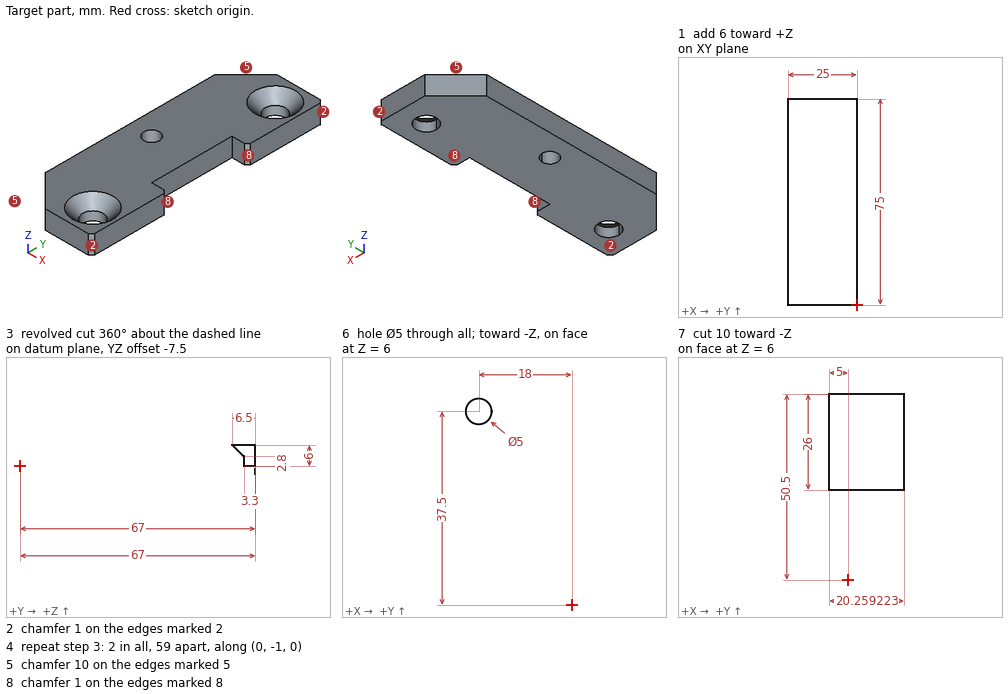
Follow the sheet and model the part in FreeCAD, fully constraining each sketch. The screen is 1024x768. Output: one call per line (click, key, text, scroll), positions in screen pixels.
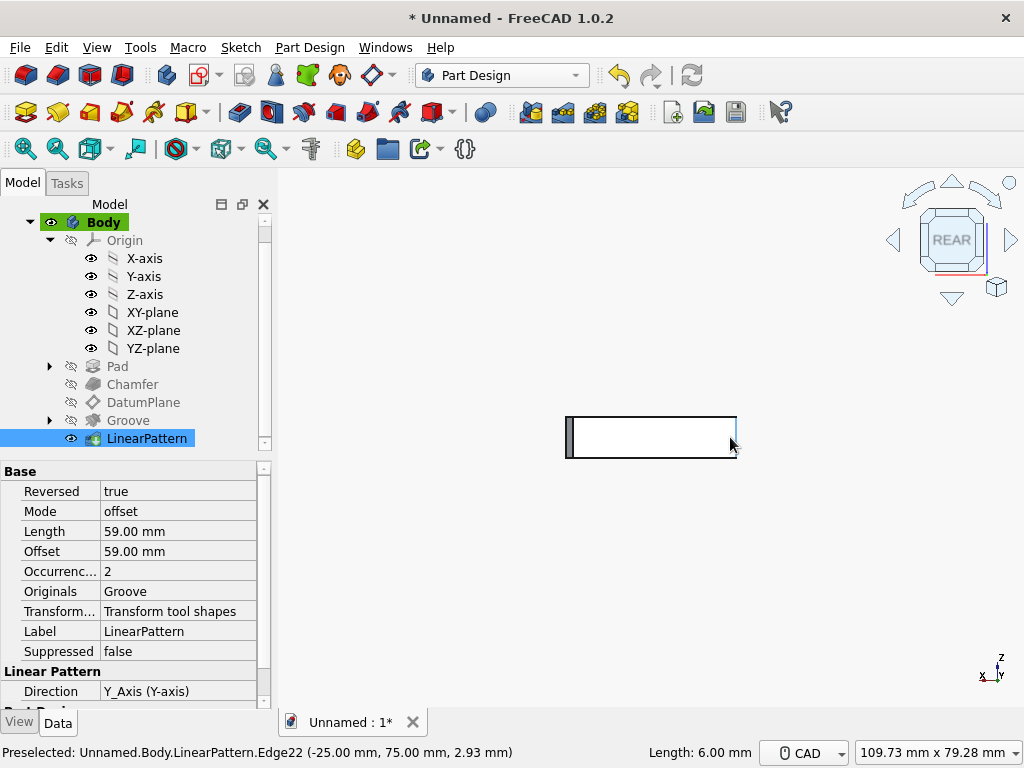
key(6)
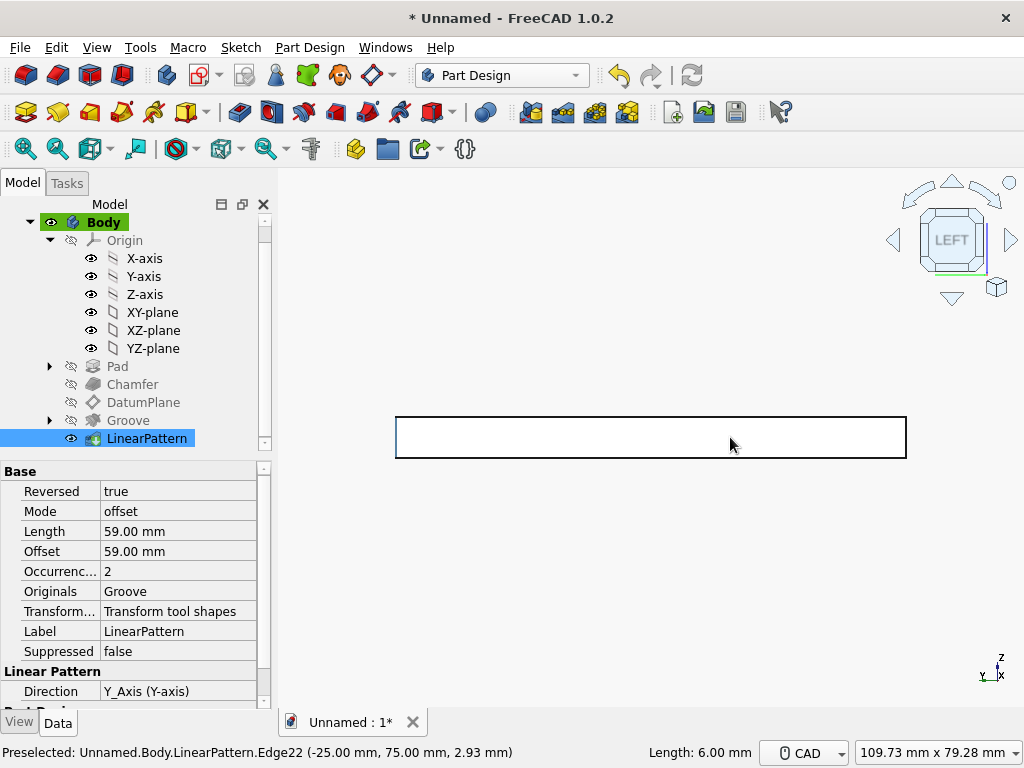
click(906, 436, ctrl)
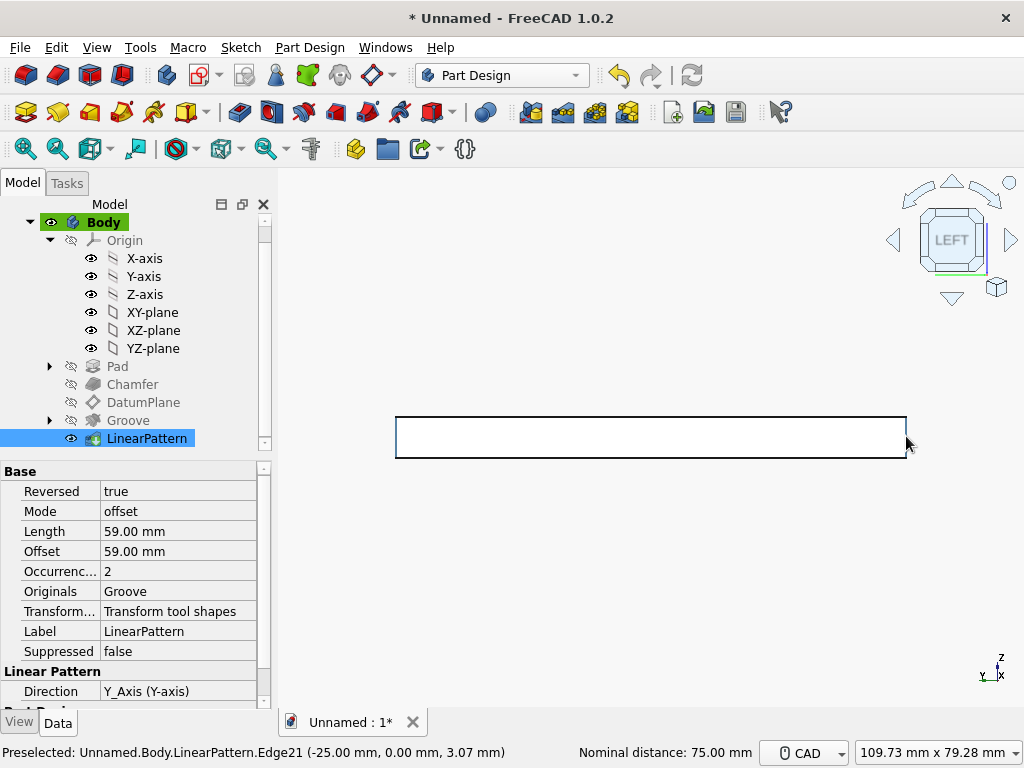
click(58, 76)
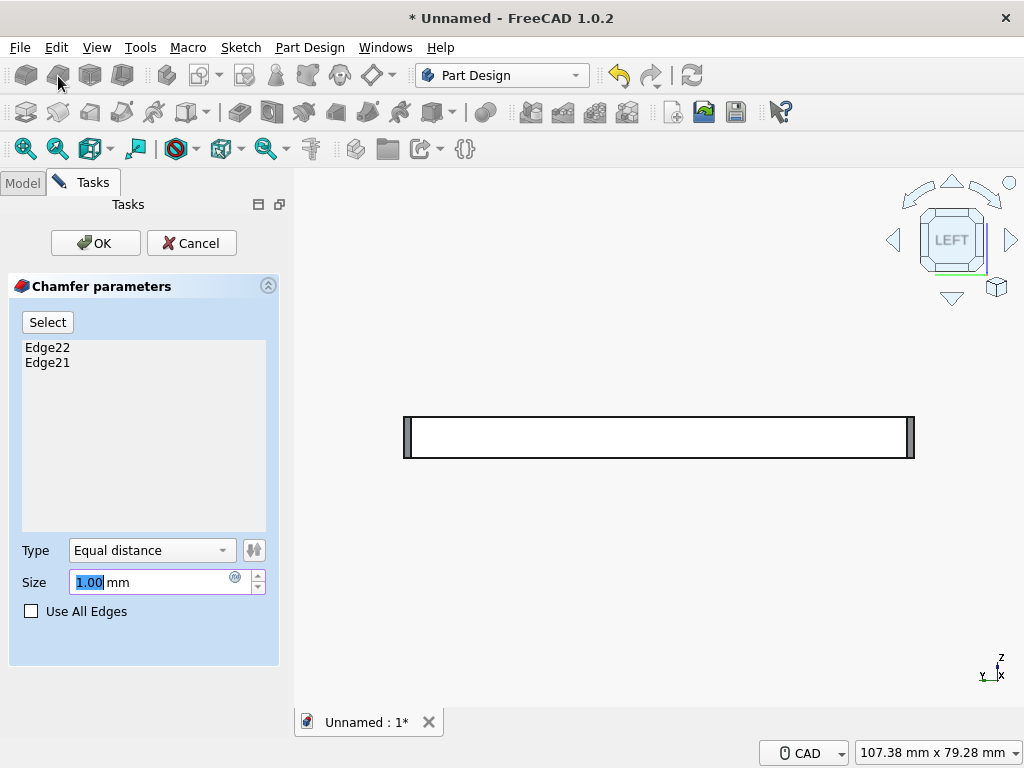
text(10)
key(Tab)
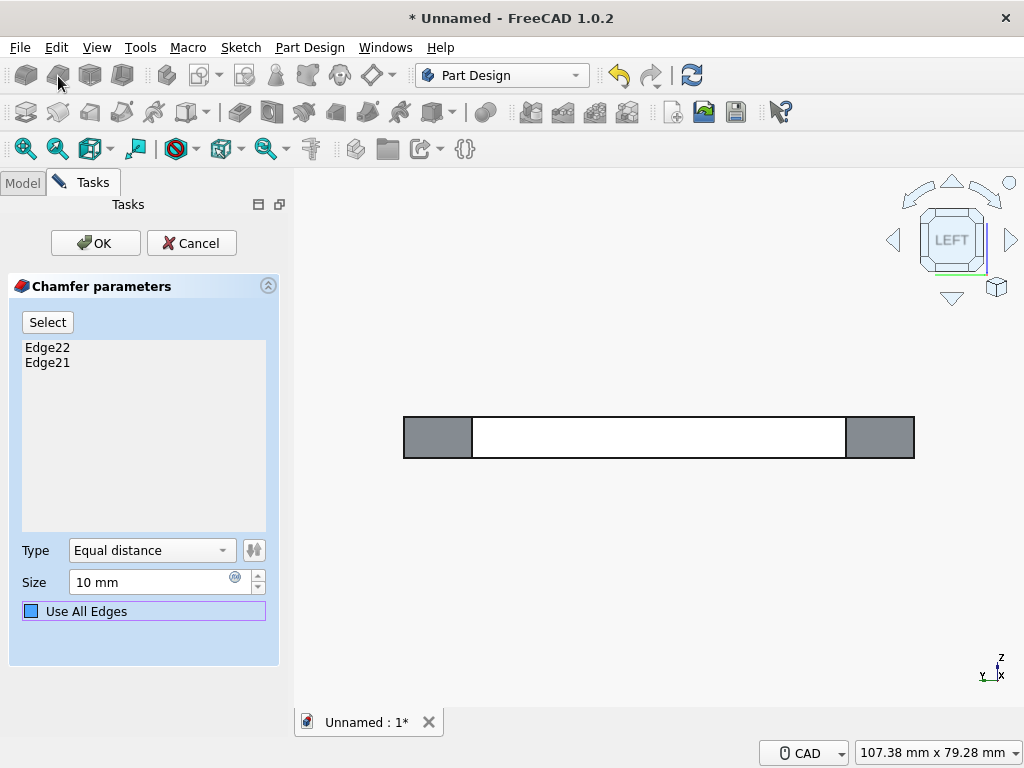
click(96, 243)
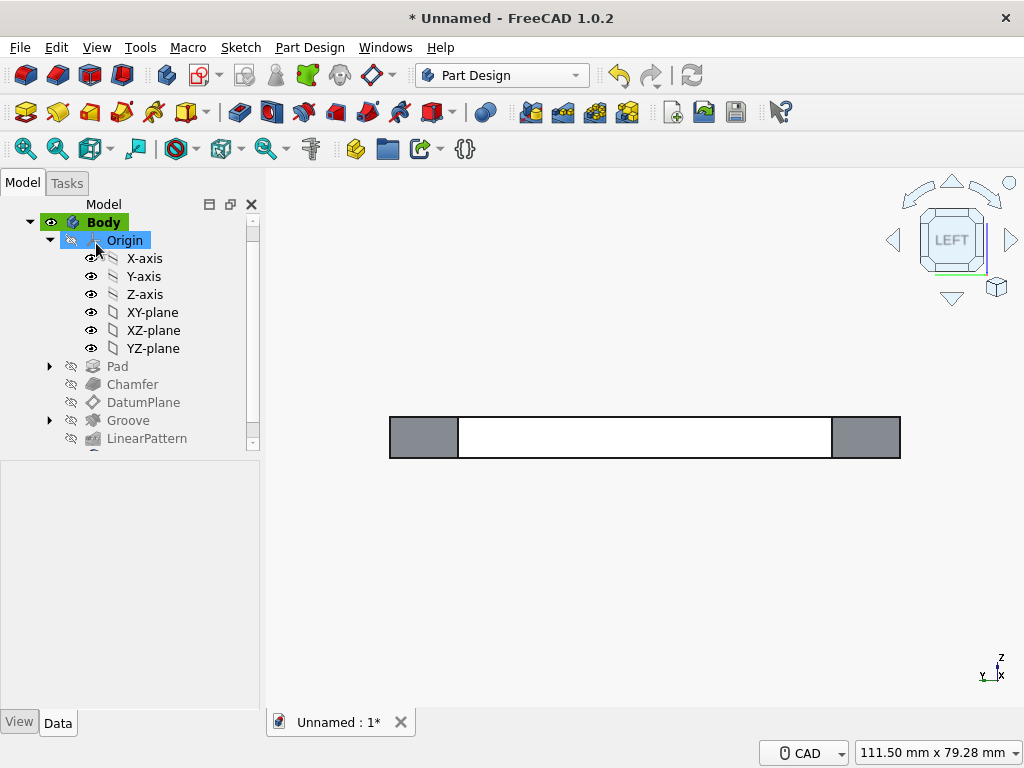
key(0)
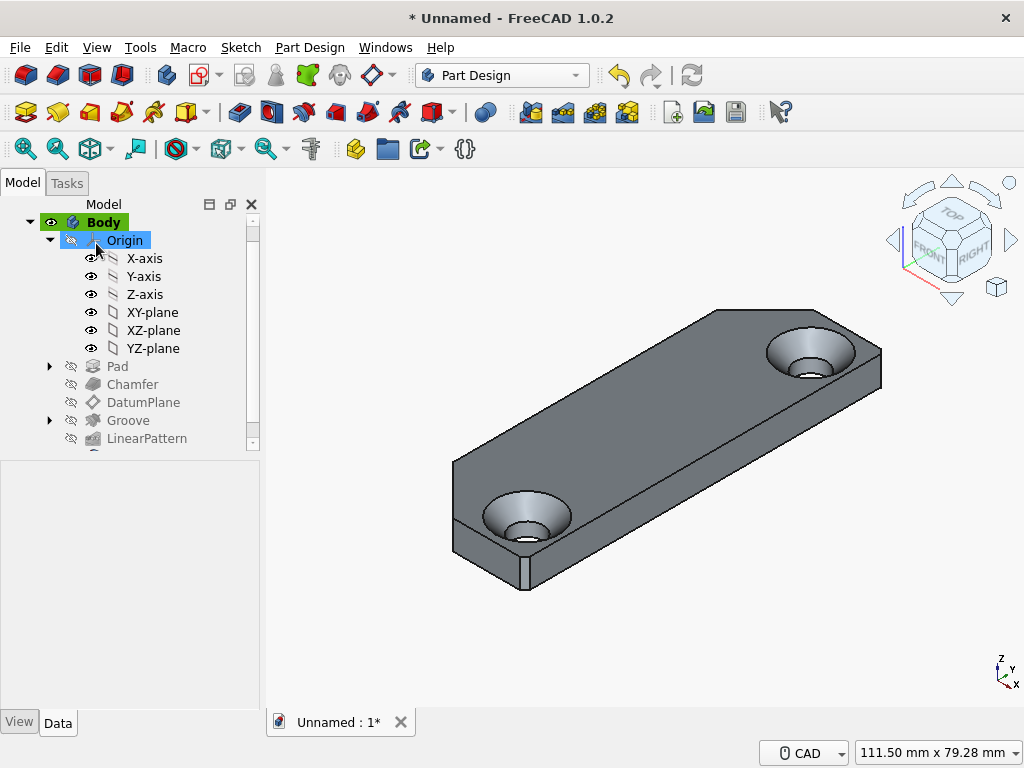
click(697, 390)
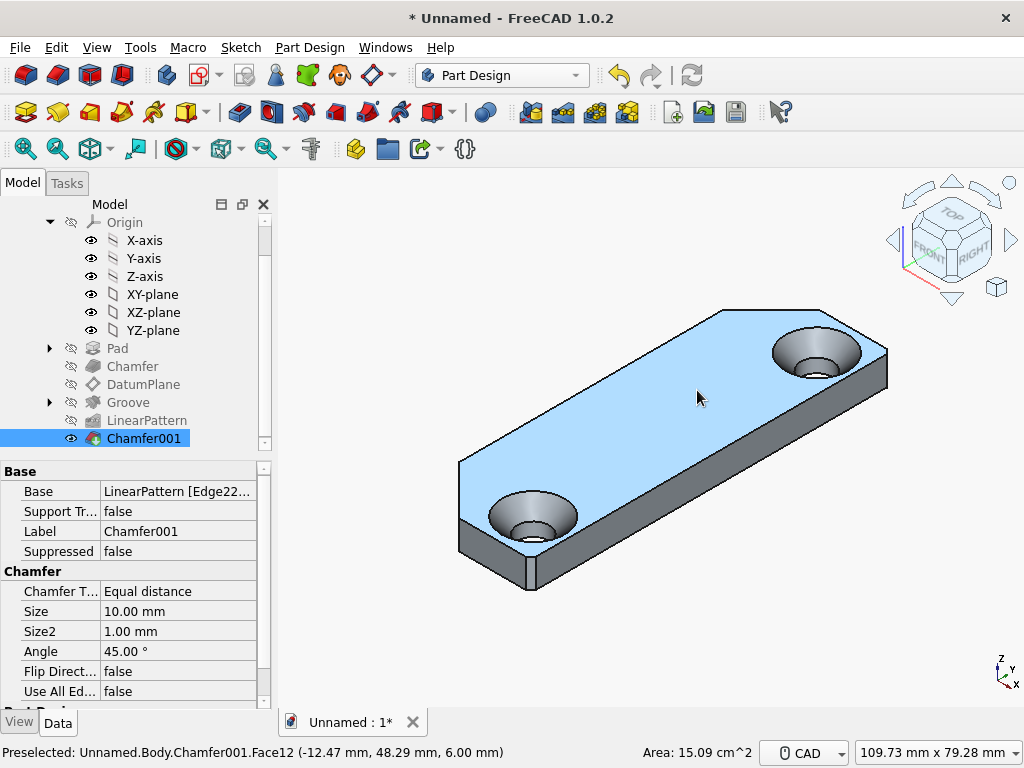
click(200, 76)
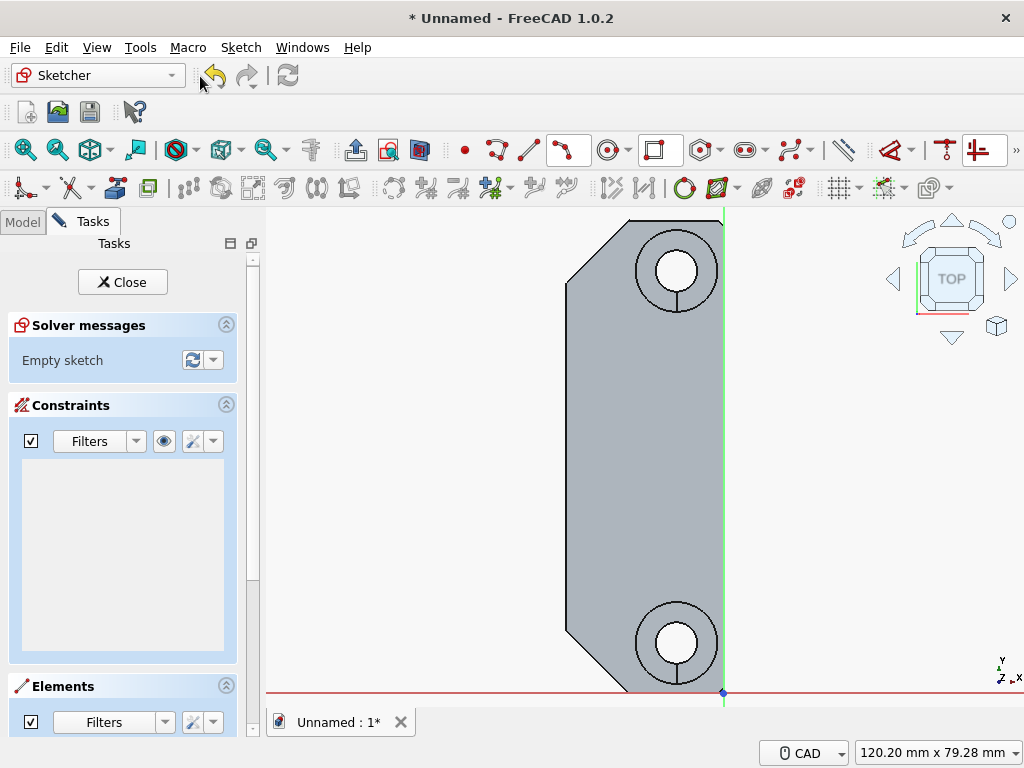
scroll(615, 457, up, 11)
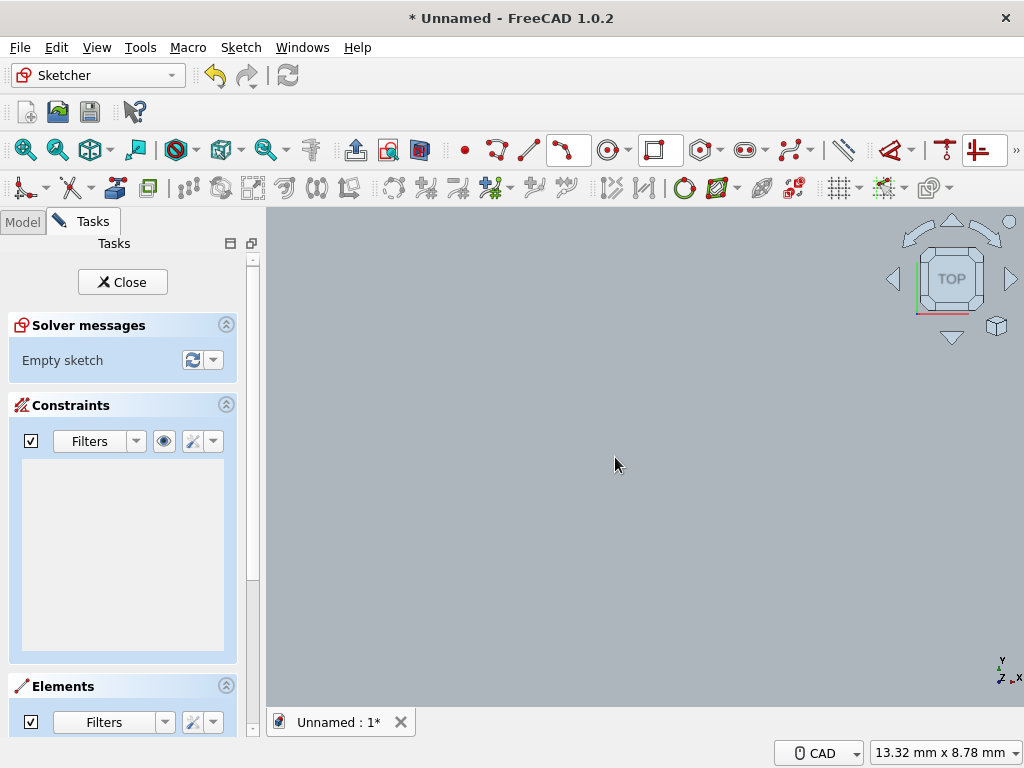
click(608, 150)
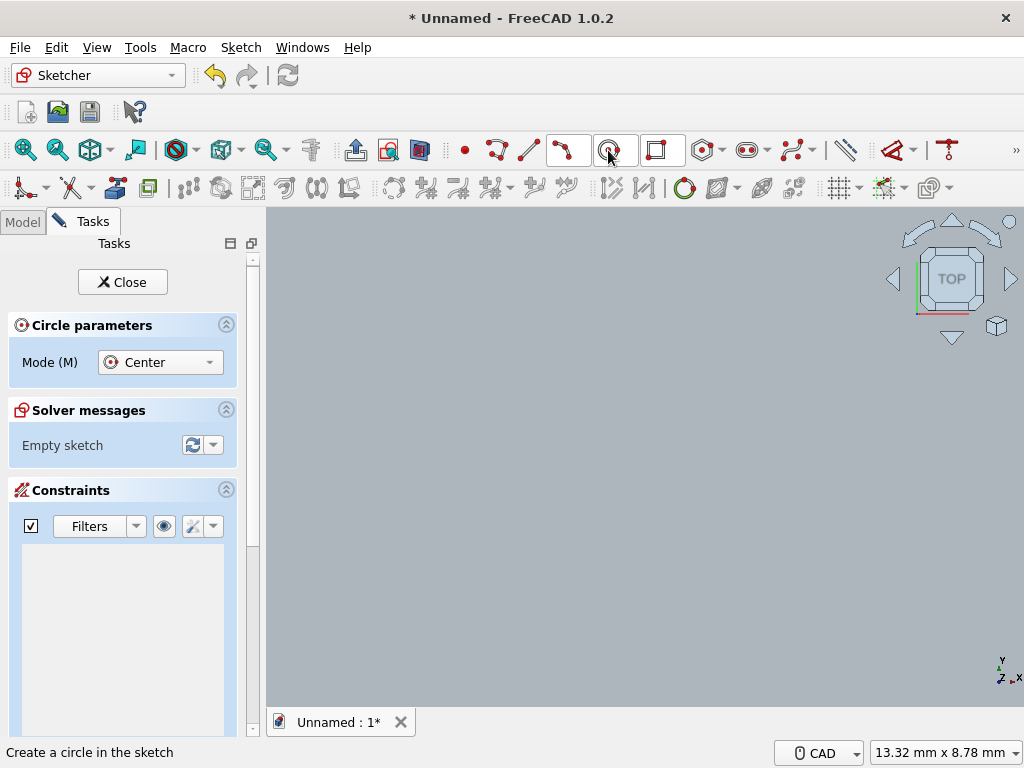
click(569, 453)
click(670, 352)
key(Escape)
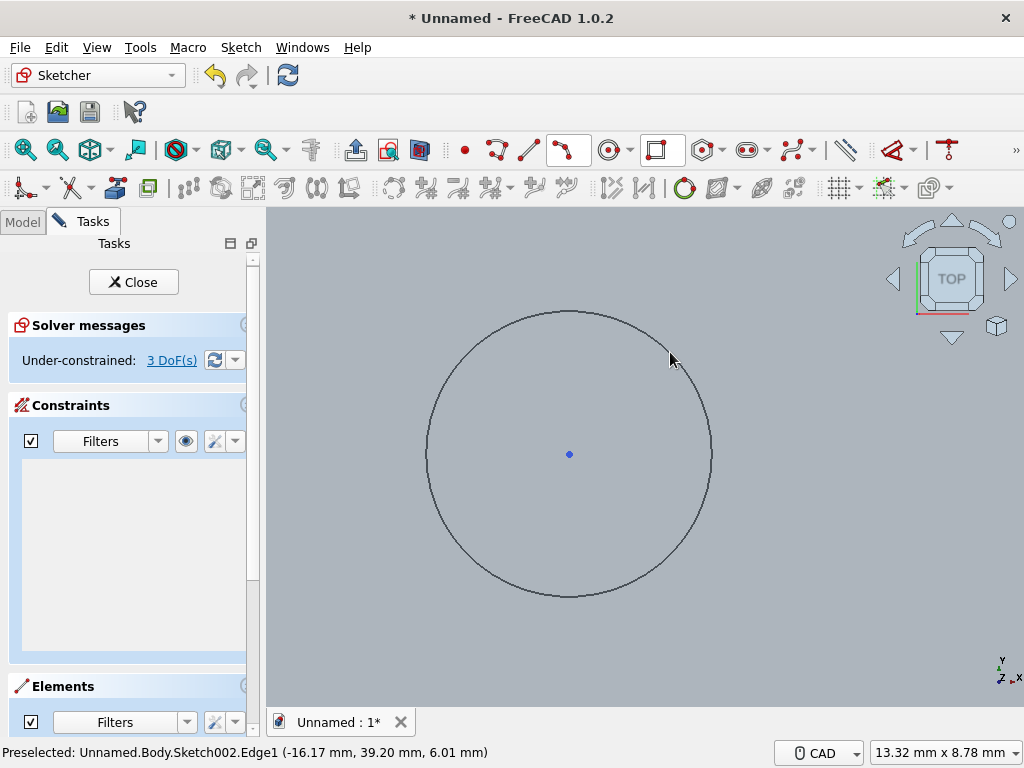
click(892, 150)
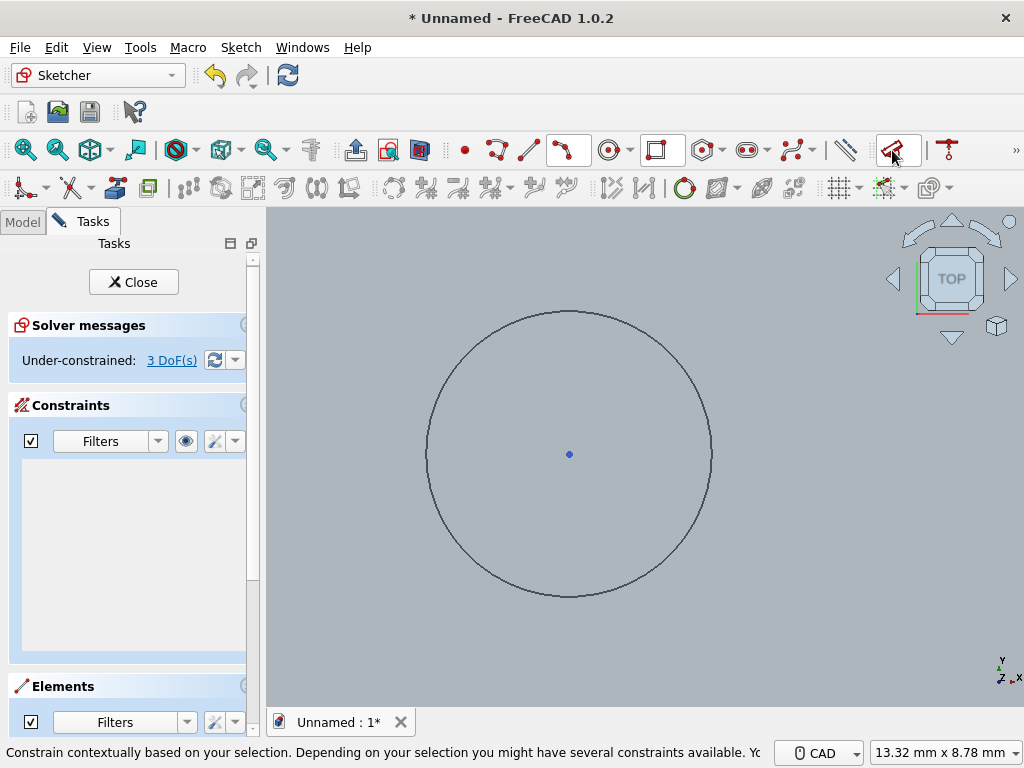
click(670, 353)
click(693, 330)